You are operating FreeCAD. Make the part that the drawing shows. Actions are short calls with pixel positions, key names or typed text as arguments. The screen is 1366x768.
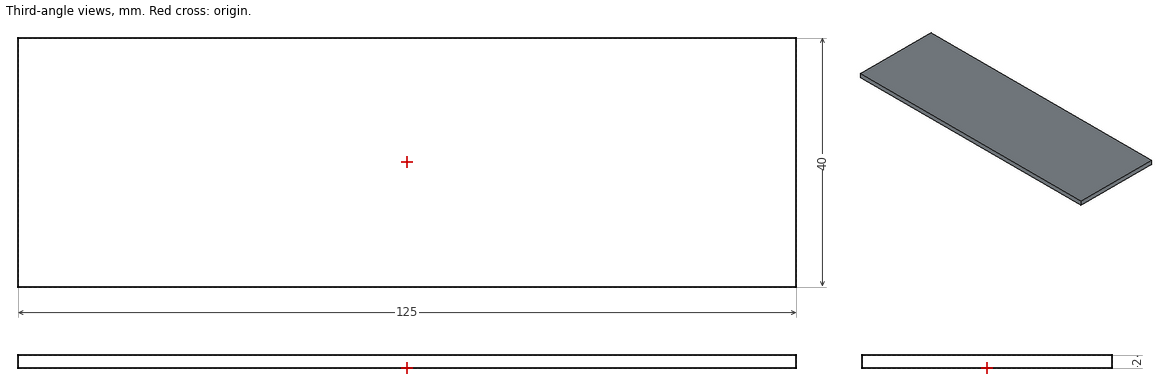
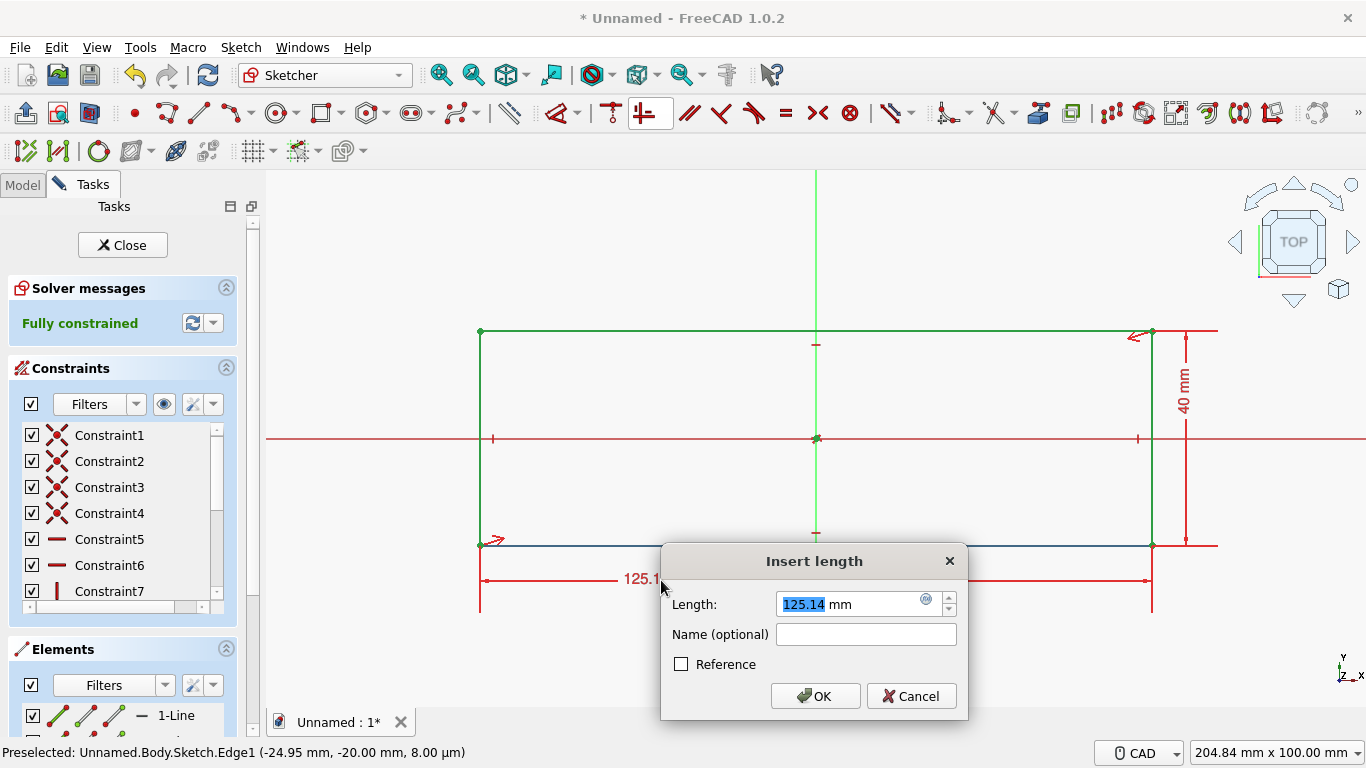
text(125)
key(Return)
key(Escape)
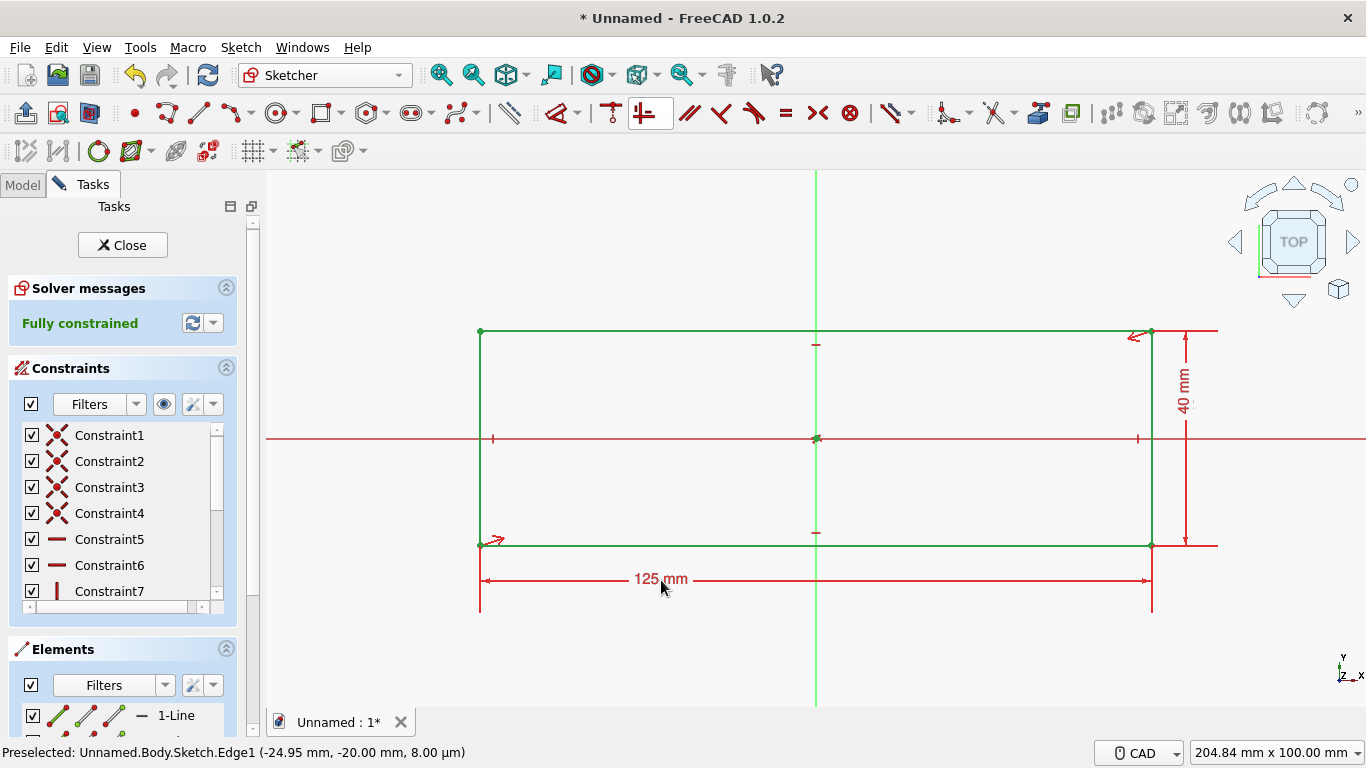
click(123, 245)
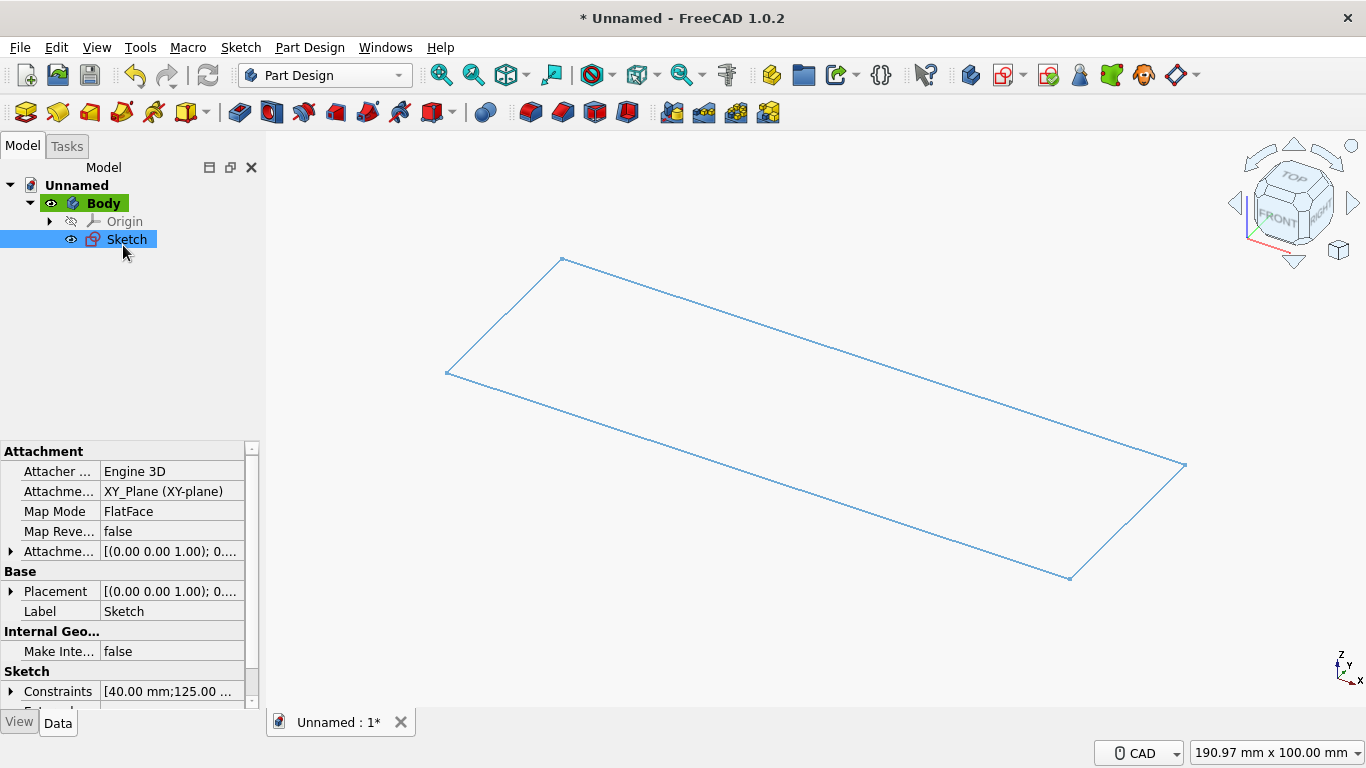
click(26, 112)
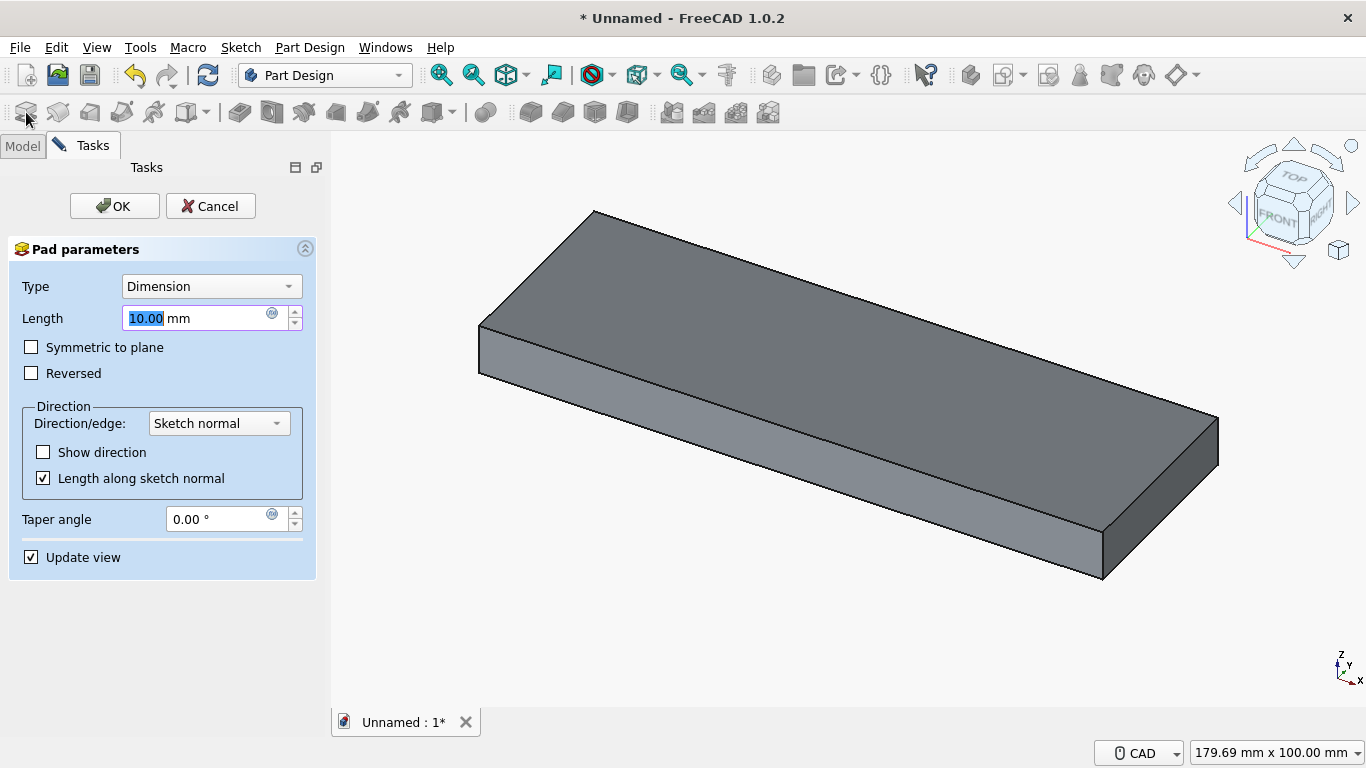
text(2)
key(Tab)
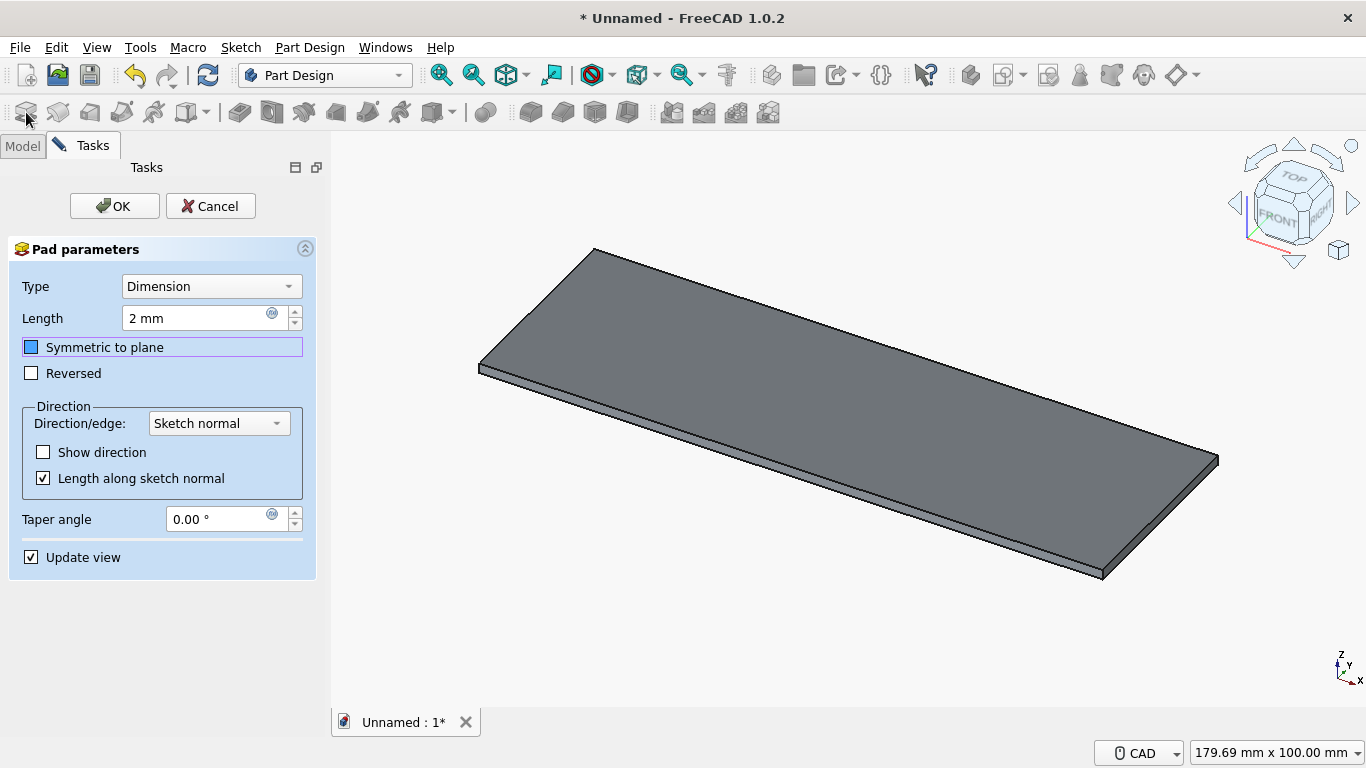
click(115, 206)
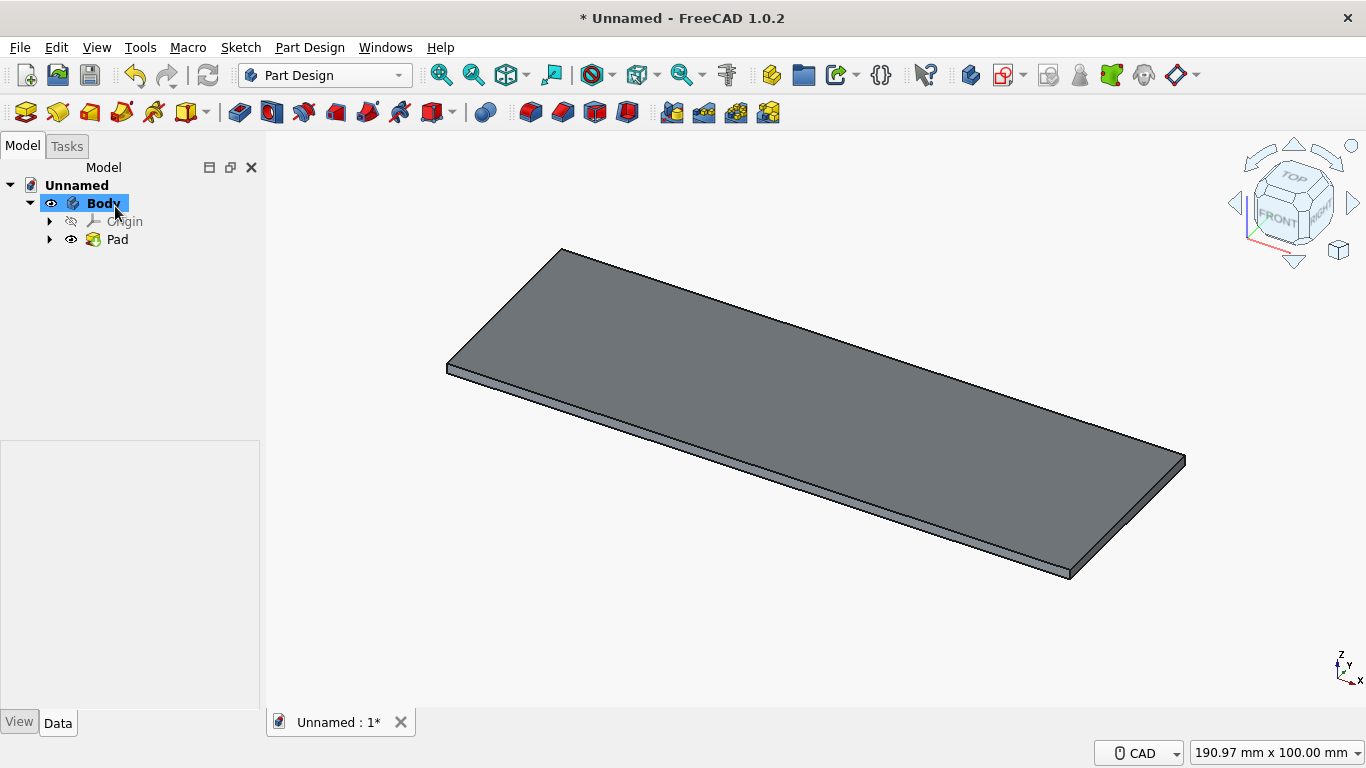
key(0)